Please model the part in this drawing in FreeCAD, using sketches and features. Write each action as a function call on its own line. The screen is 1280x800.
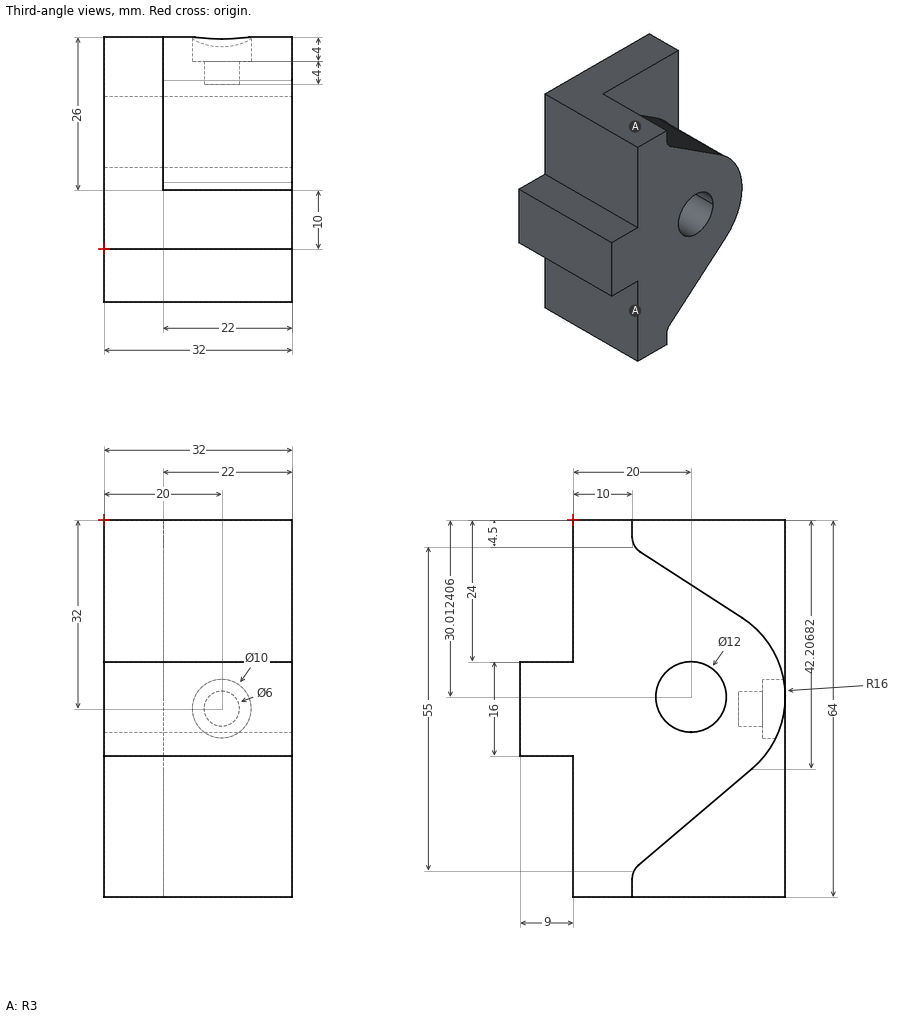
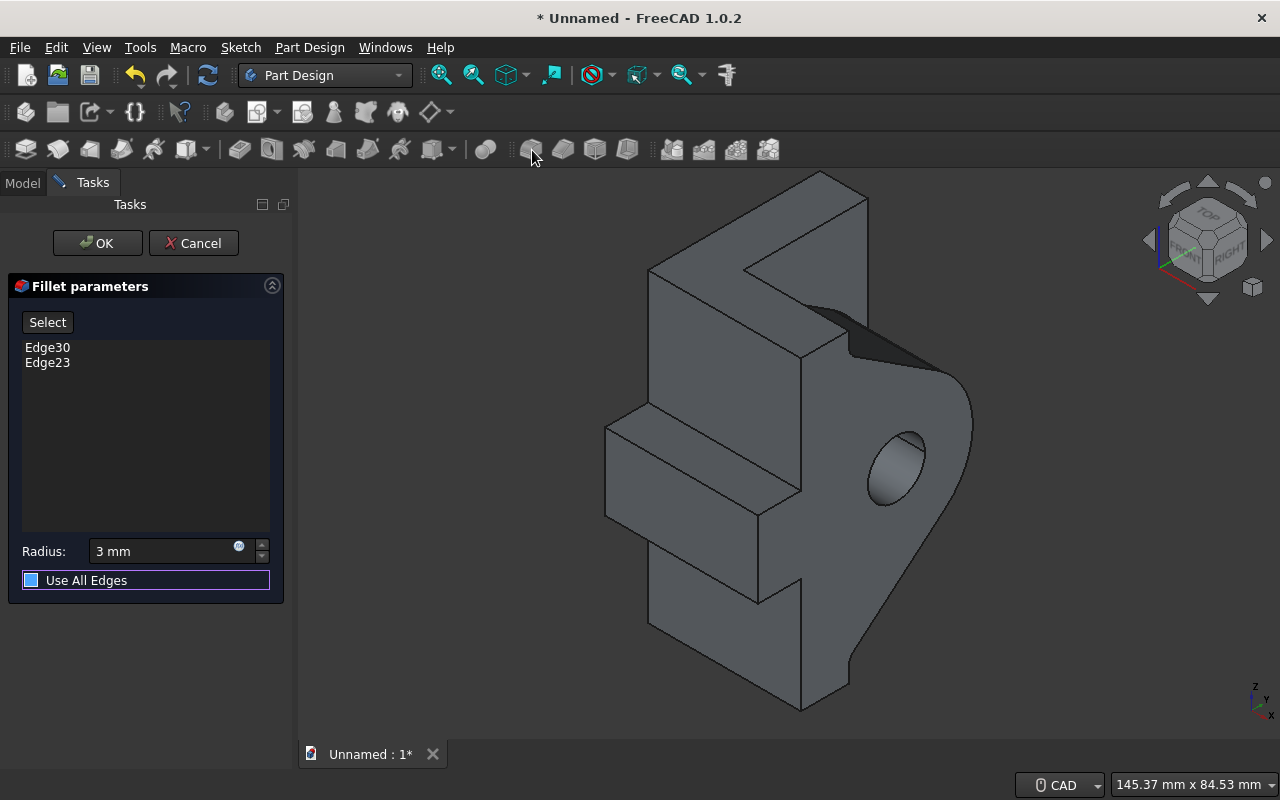
click(98, 243)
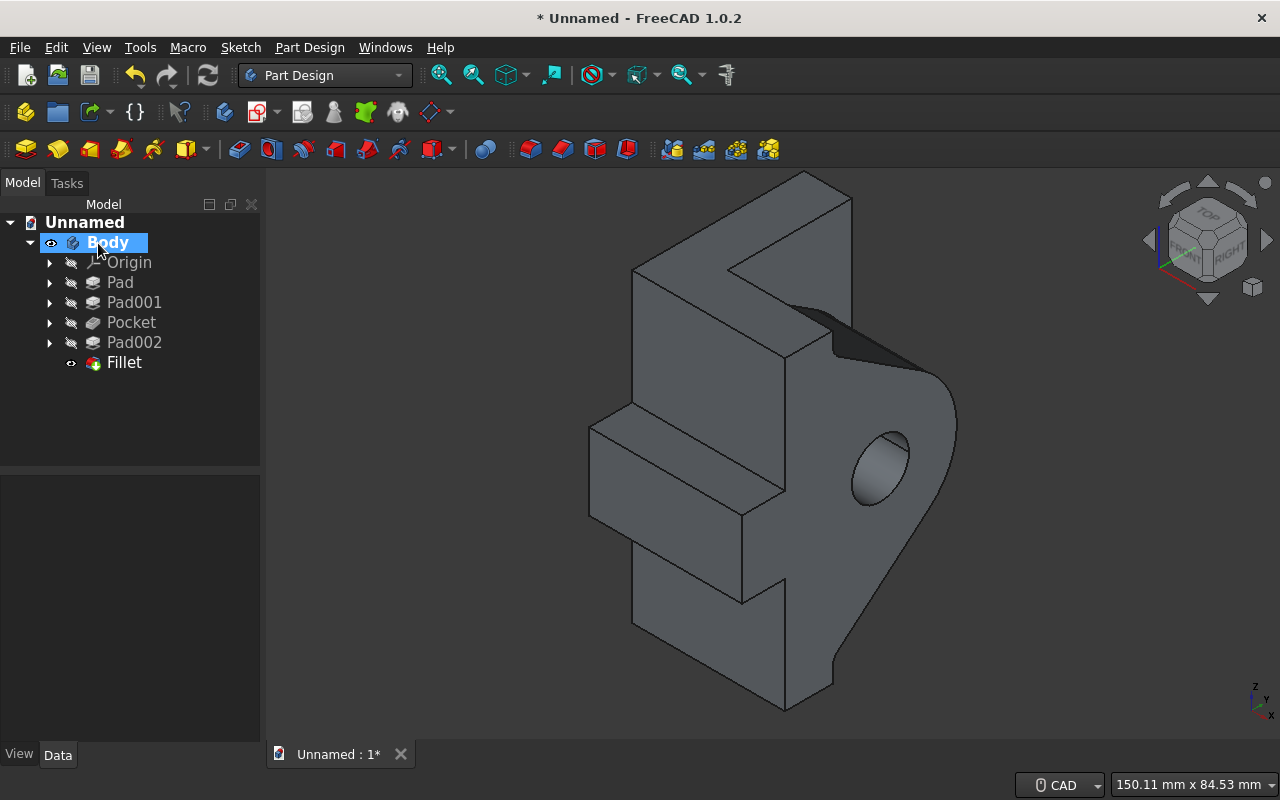
key(4)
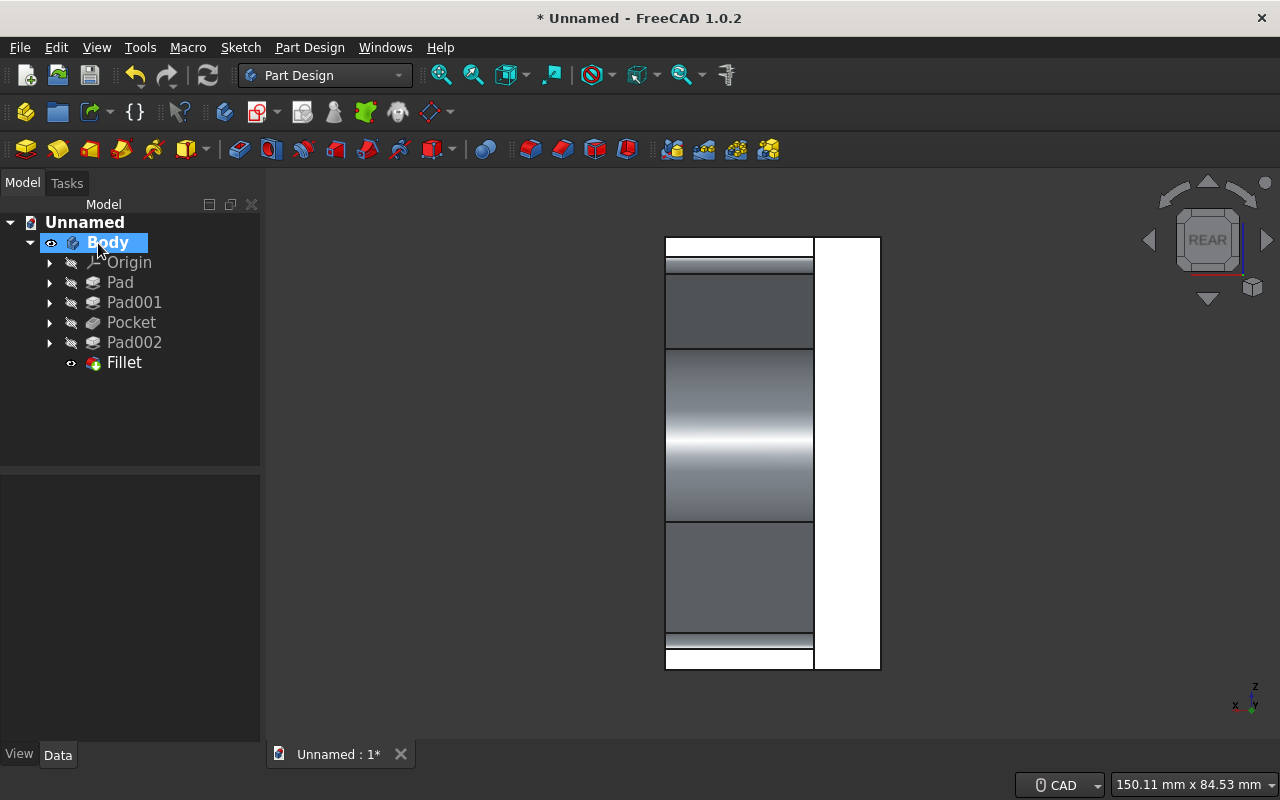
click(847, 329)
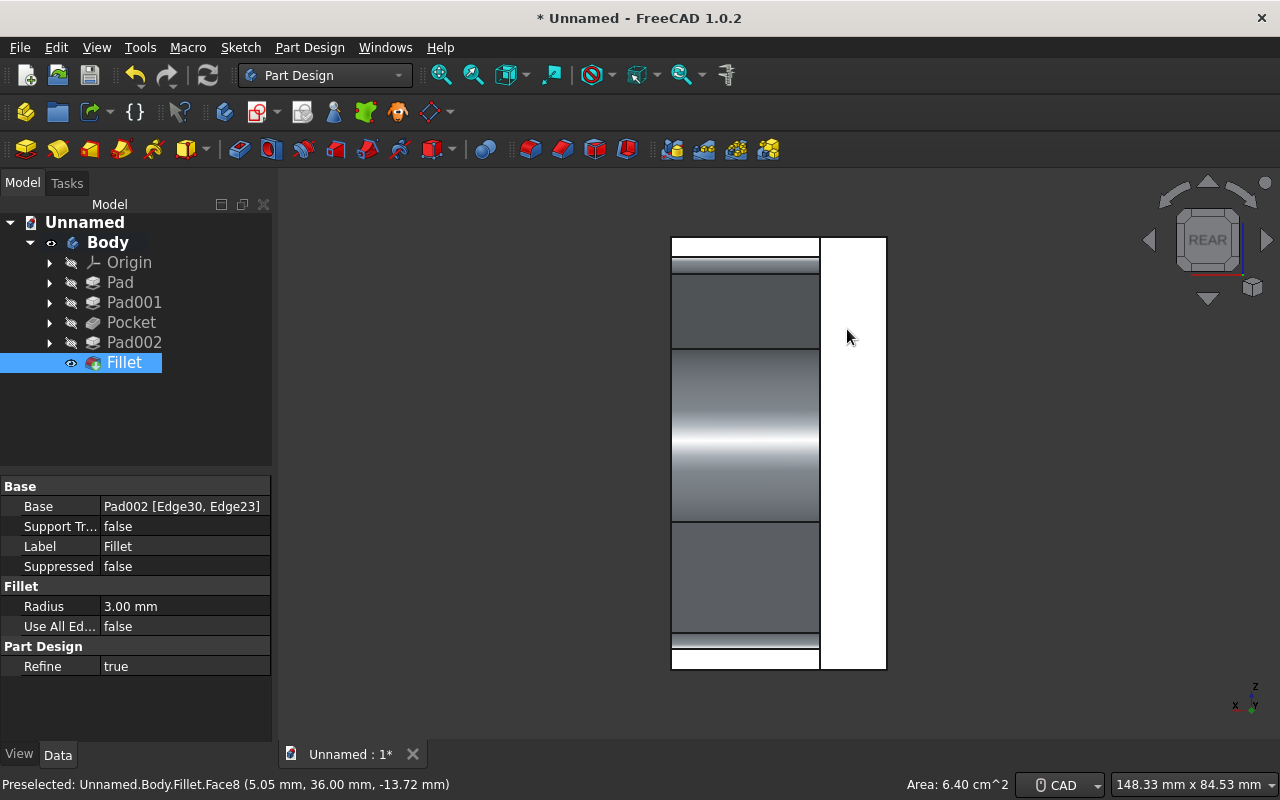
click(258, 112)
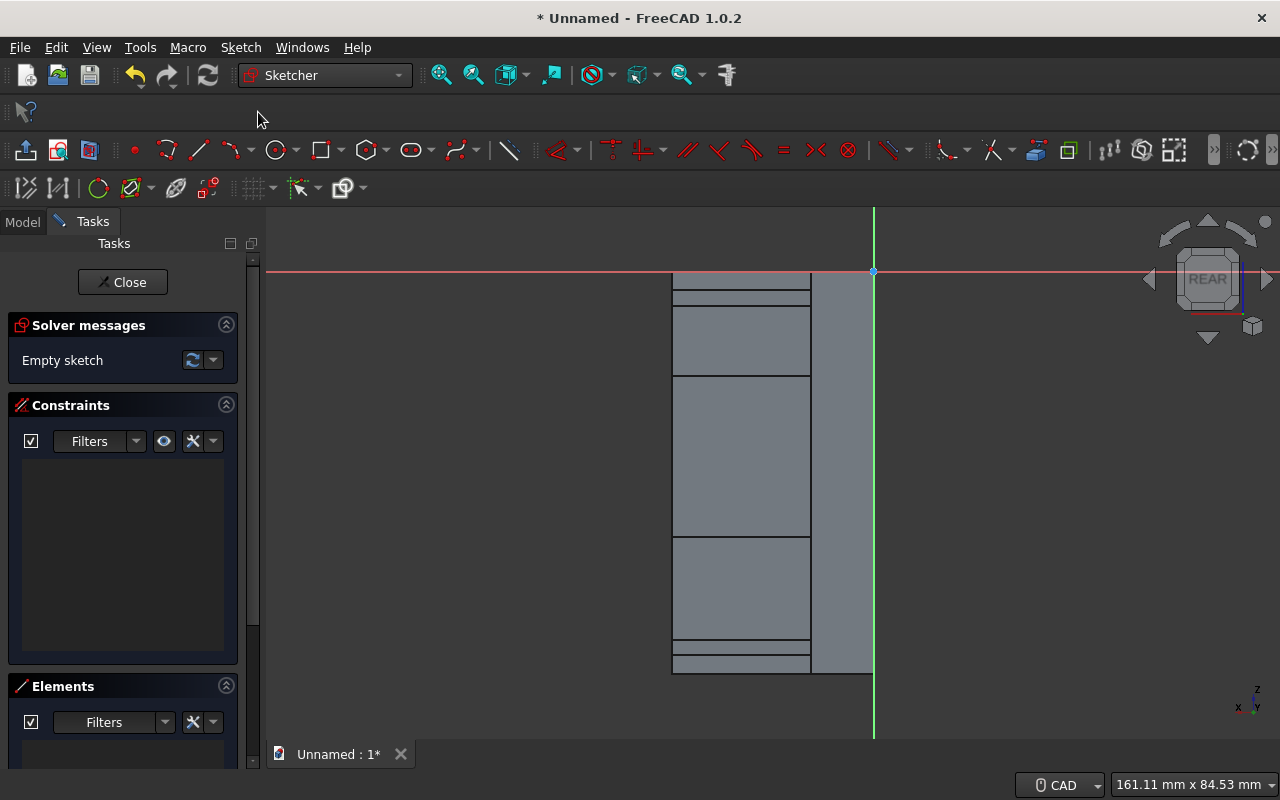
scroll(759, 473, up, 8)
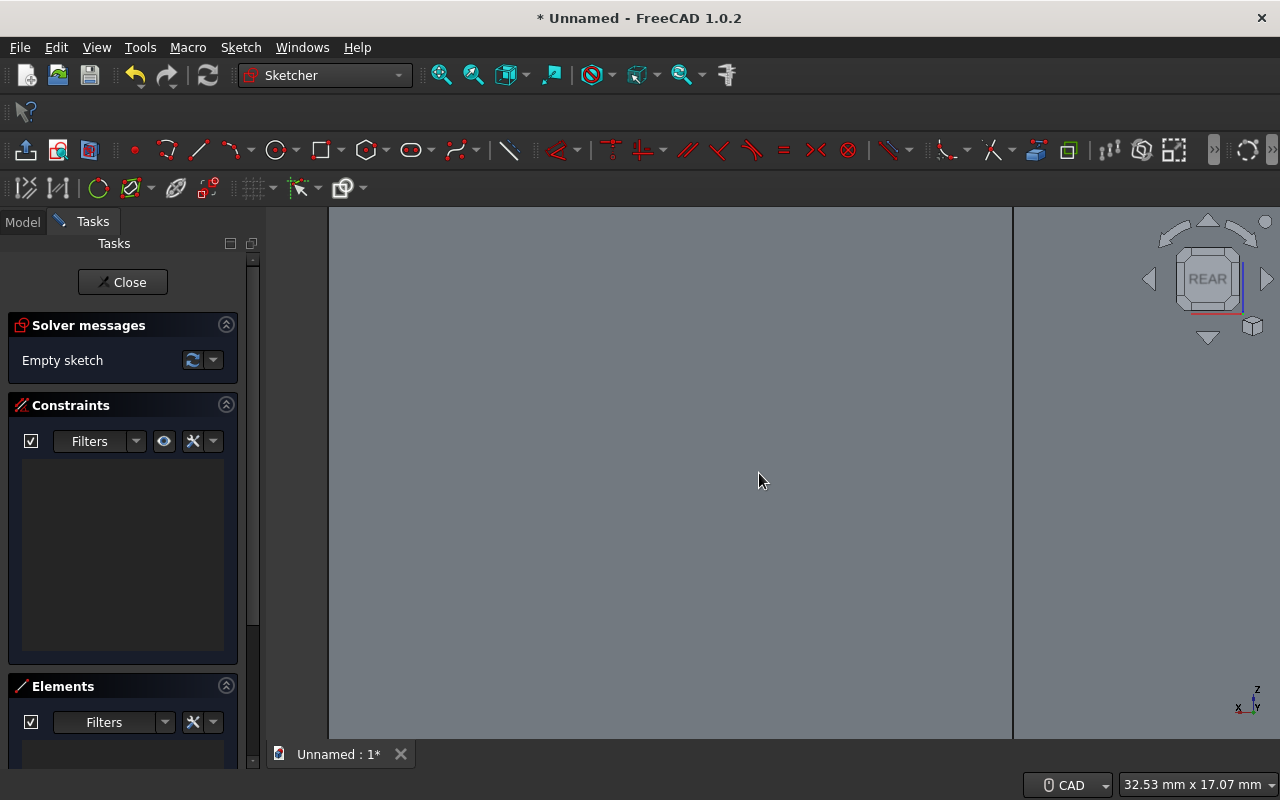
key(g)
key(c)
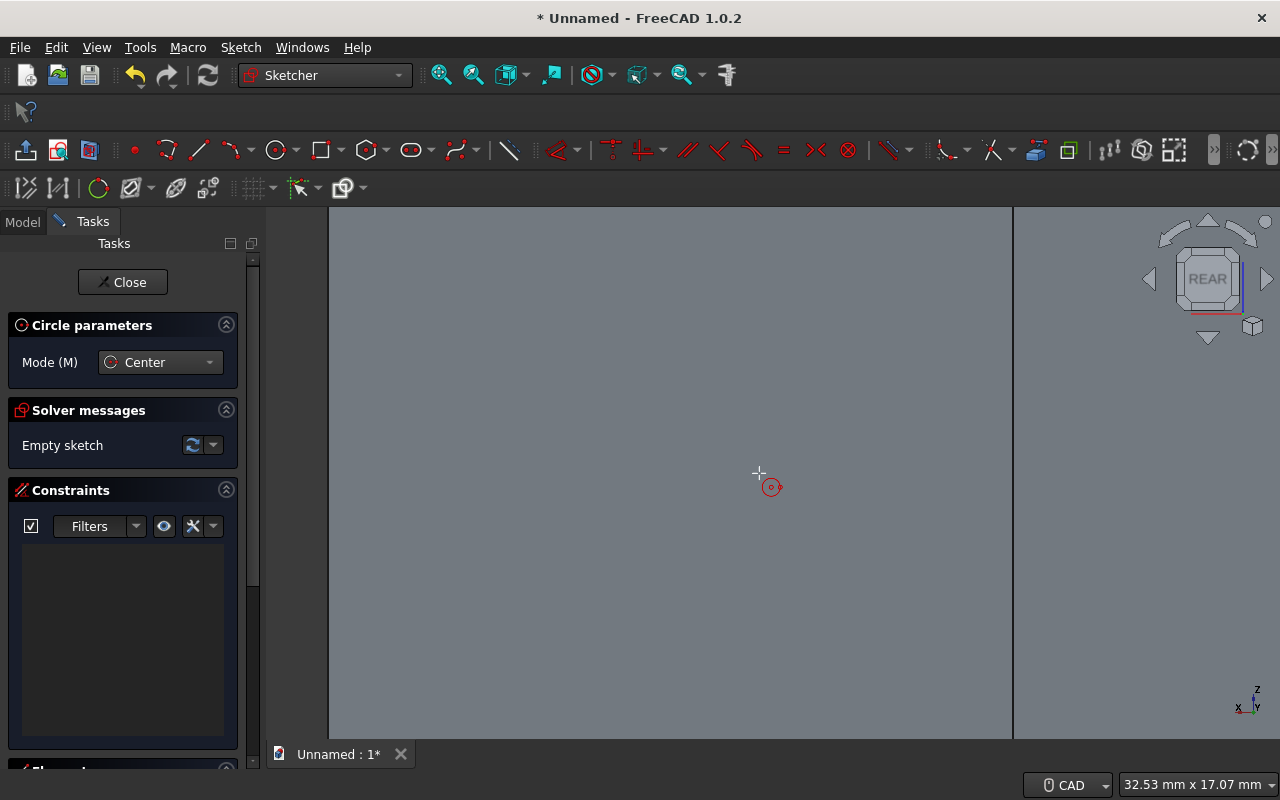
click(702, 471)
move(812, 361)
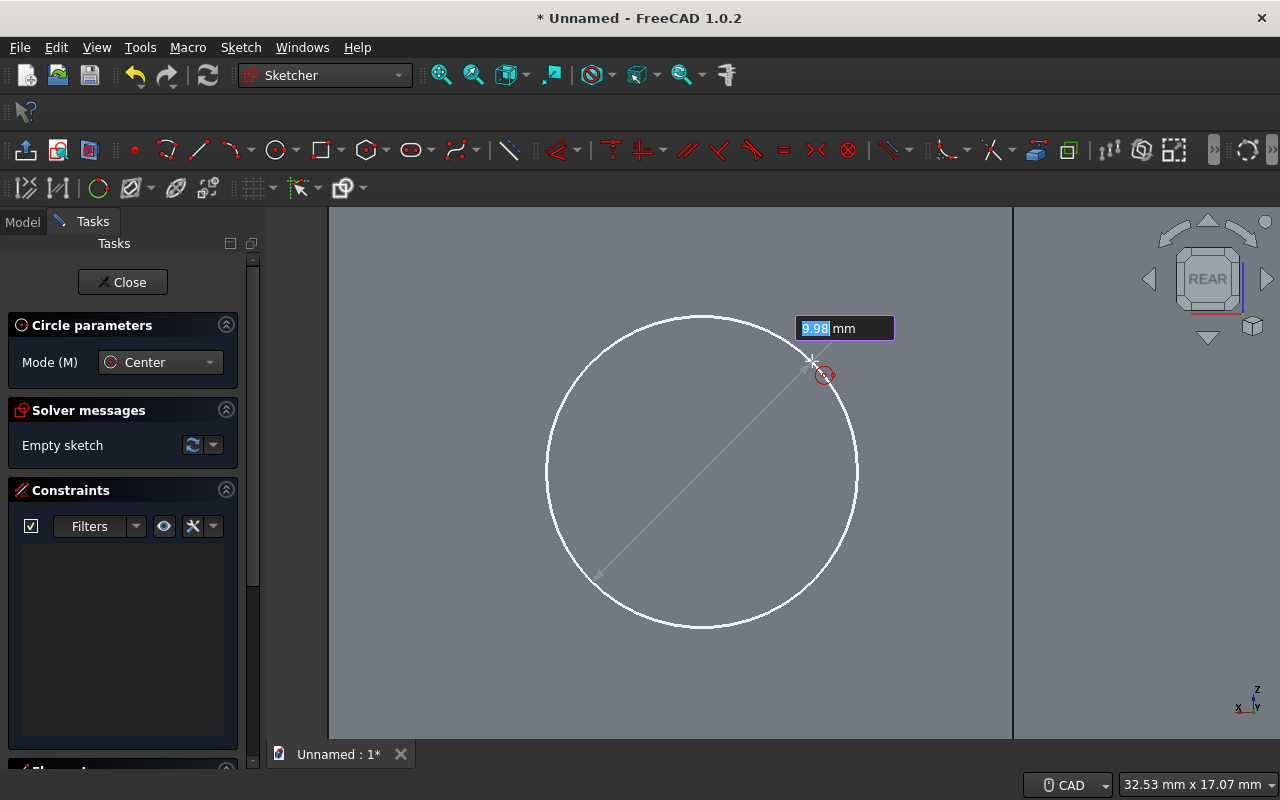
text(10)
key(Return)
key(Escape)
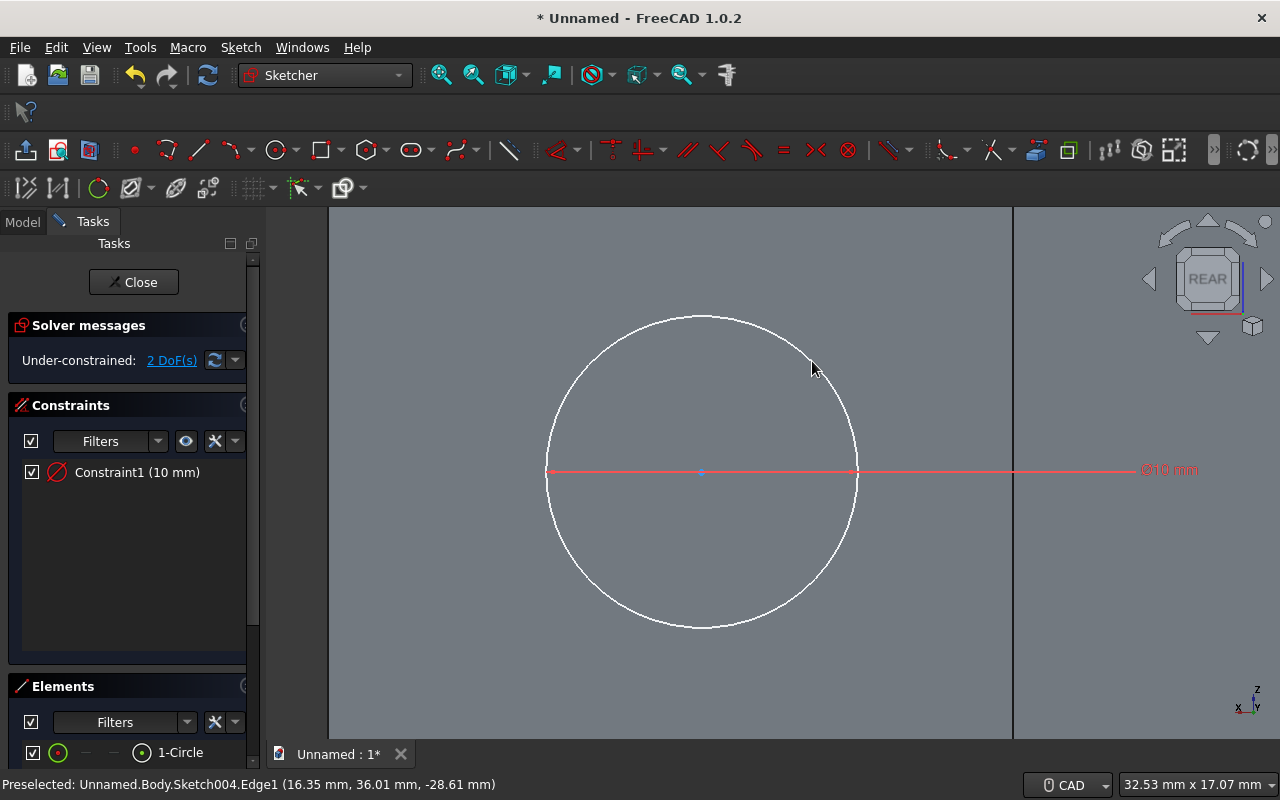
key(d)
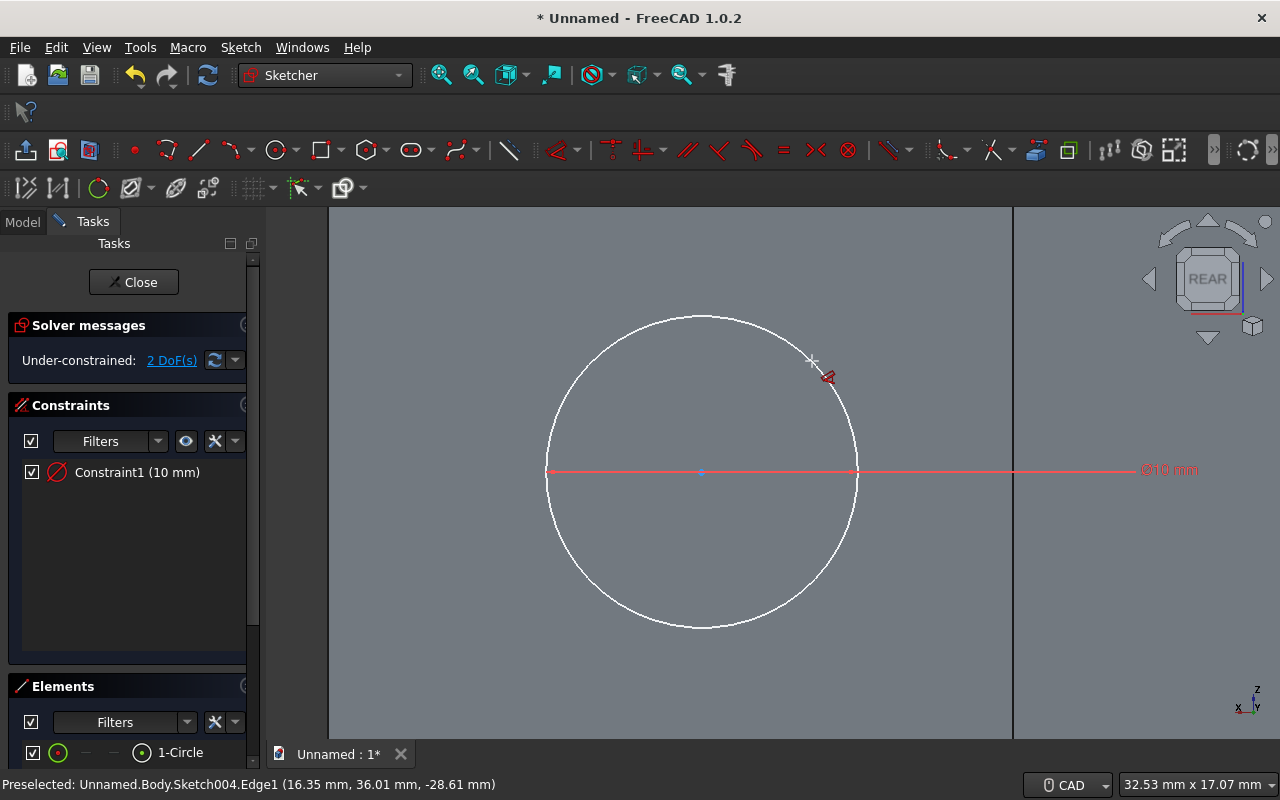
click(702, 472)
click(909, 506)